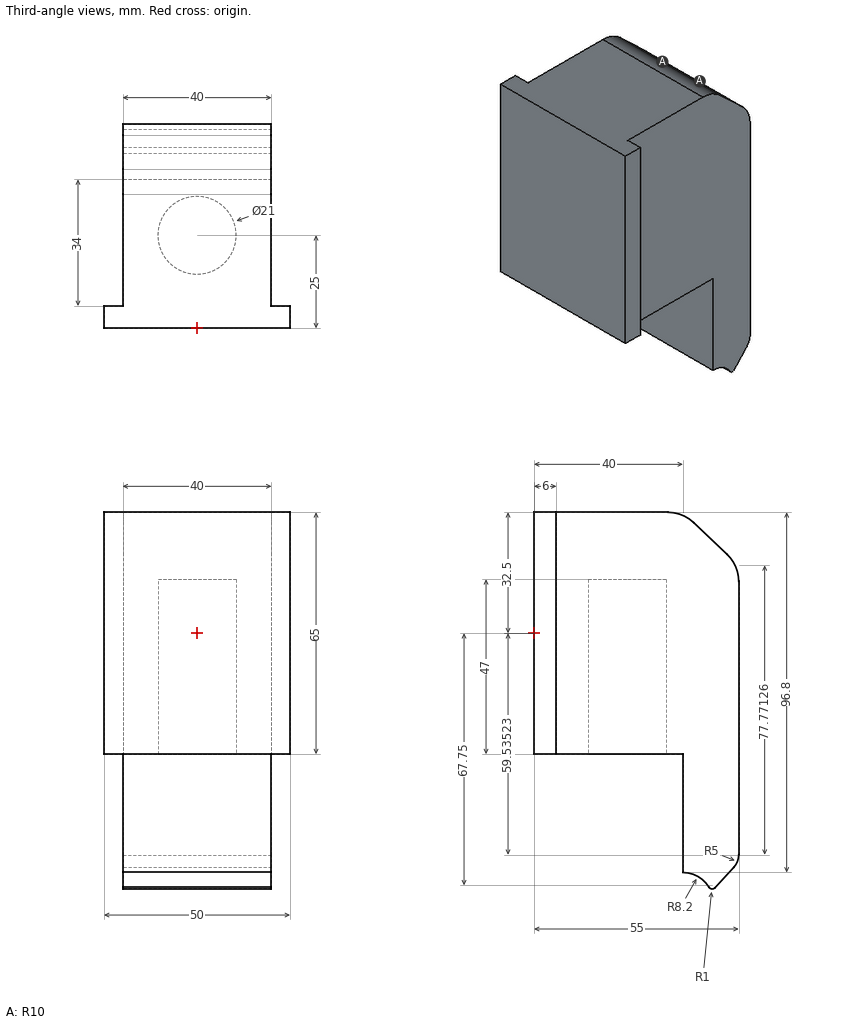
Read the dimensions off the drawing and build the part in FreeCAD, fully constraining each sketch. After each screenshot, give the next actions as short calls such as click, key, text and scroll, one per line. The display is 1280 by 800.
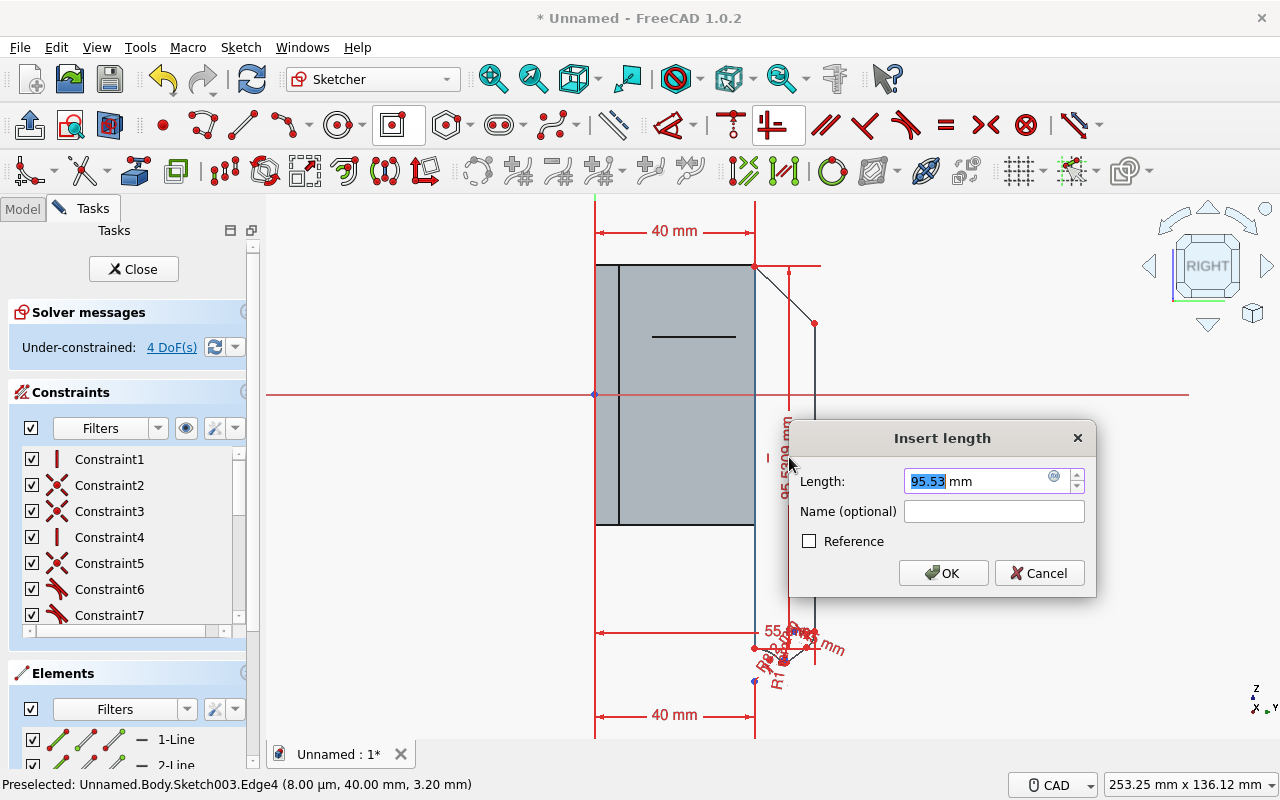
text(96.8)
key(Return)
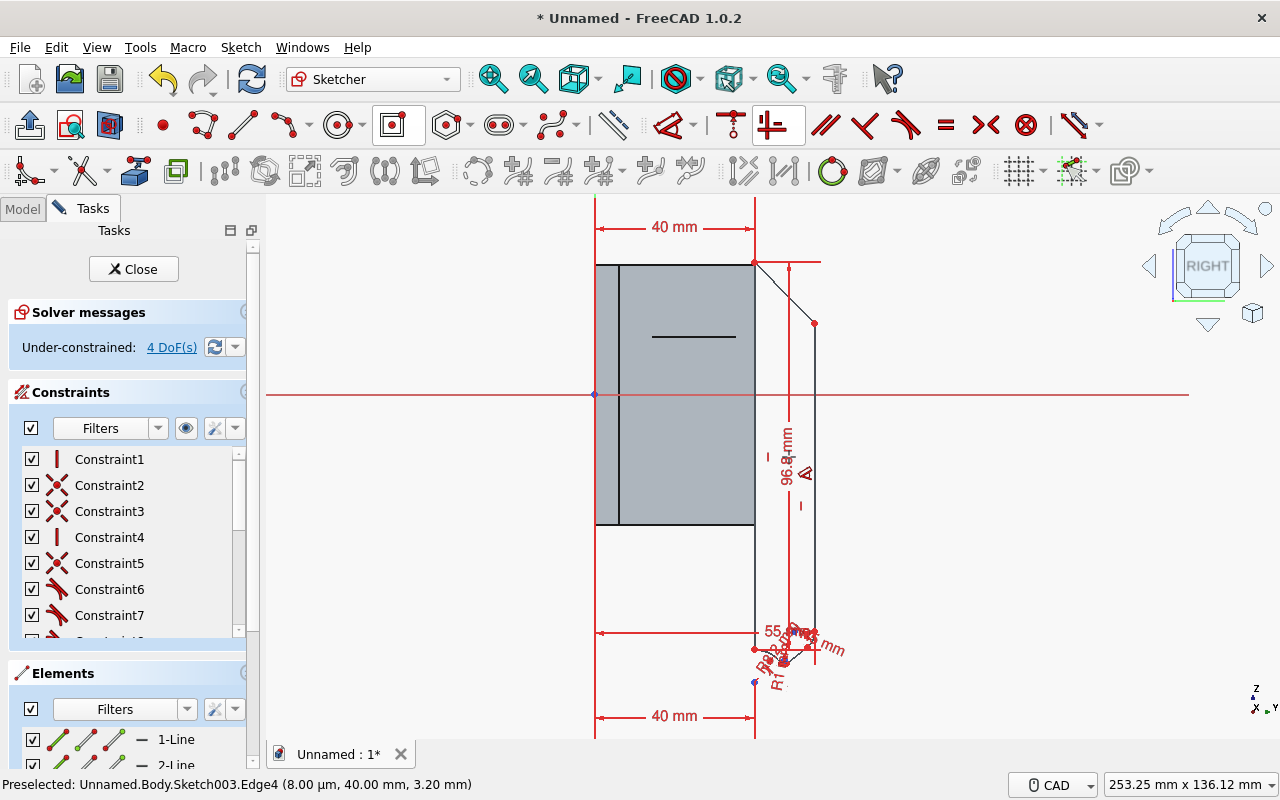
click(755, 262)
click(561, 329)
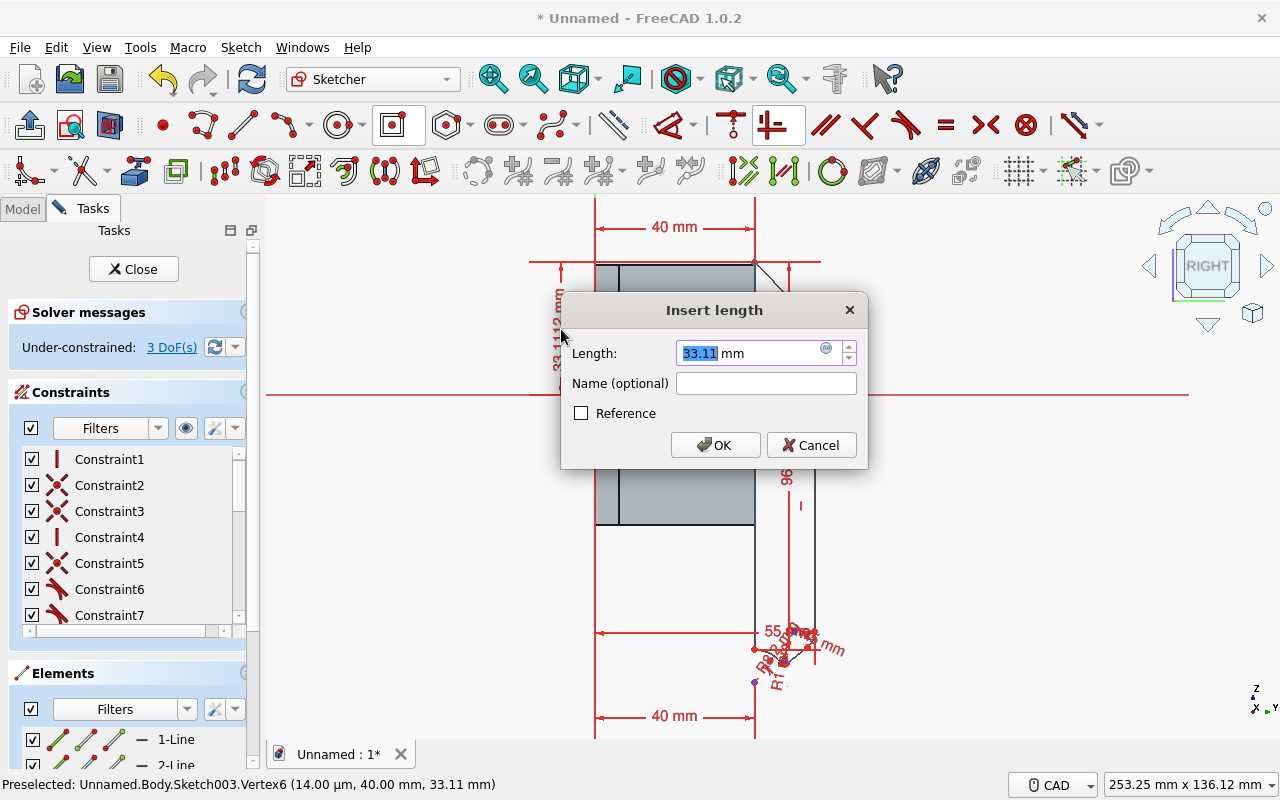
text(32.5)
key(Return)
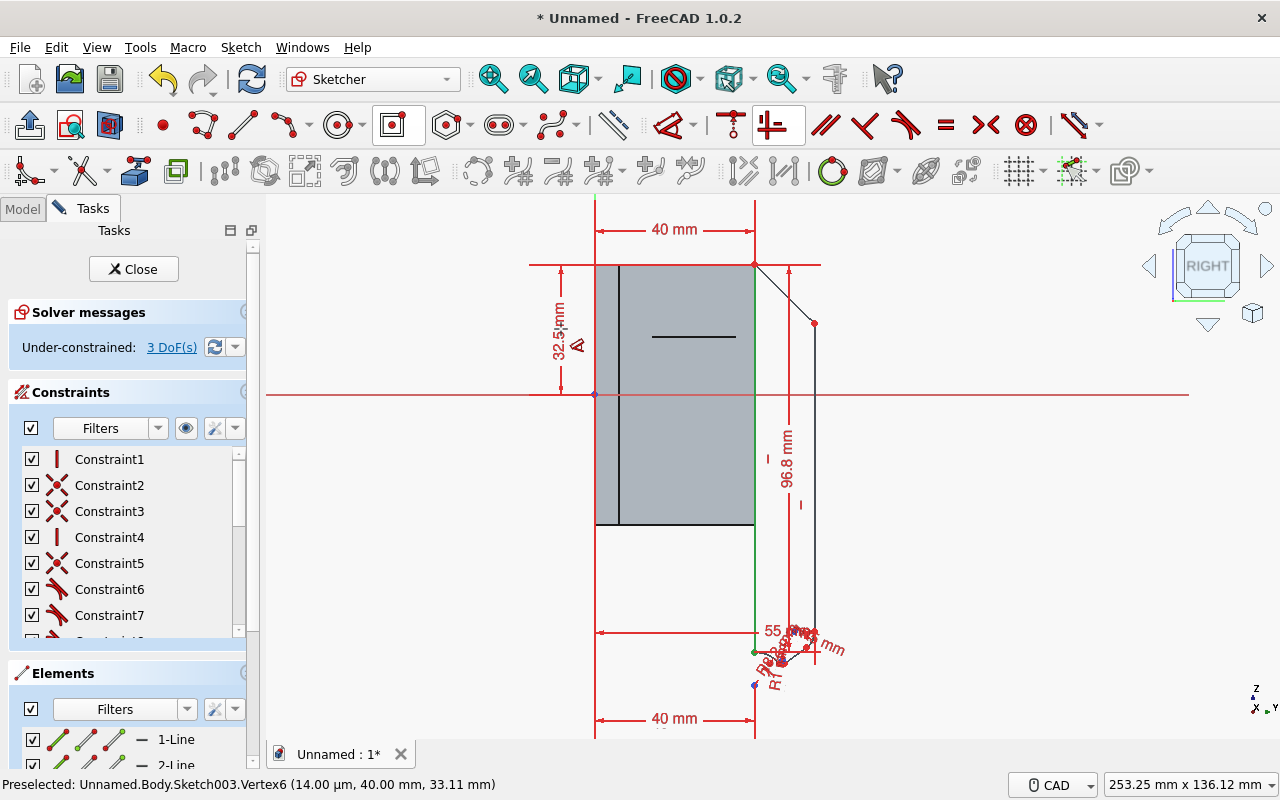
scroll(782, 661, up, 6)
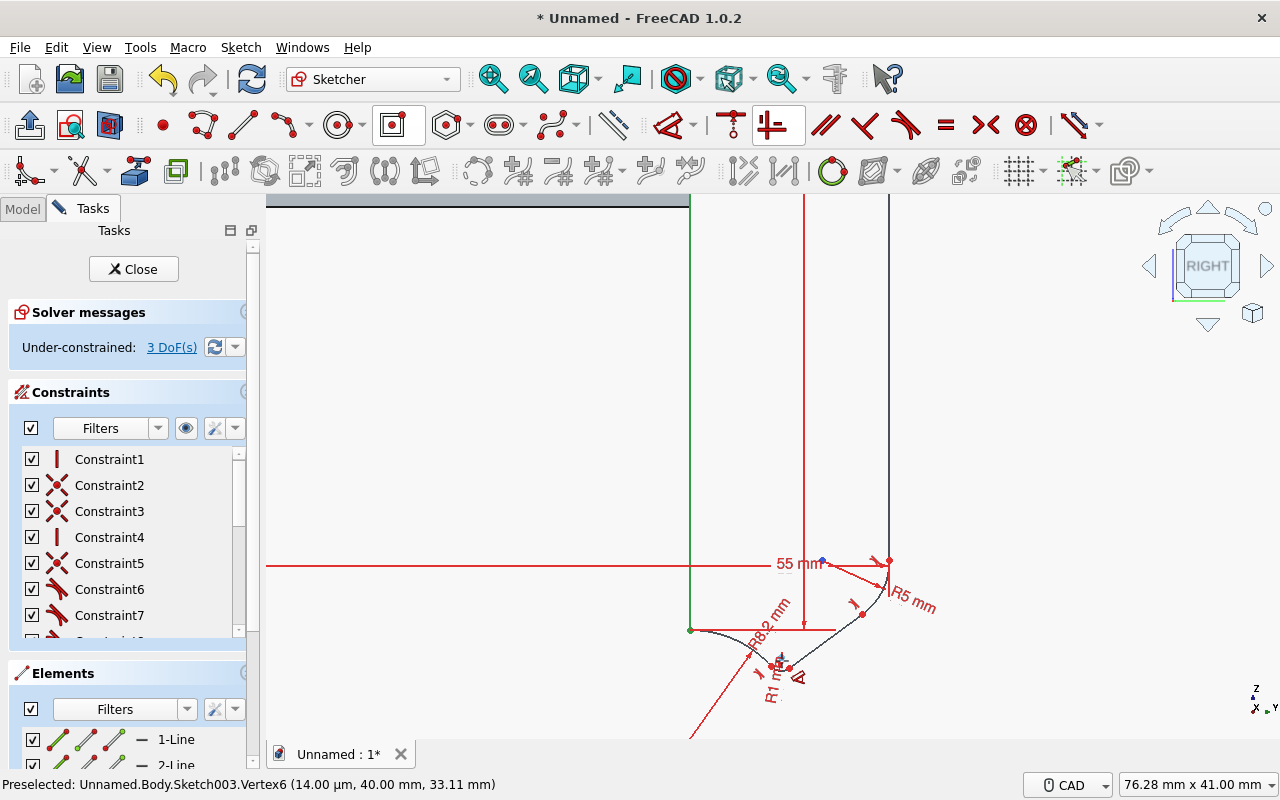
click(781, 658)
click(815, 440)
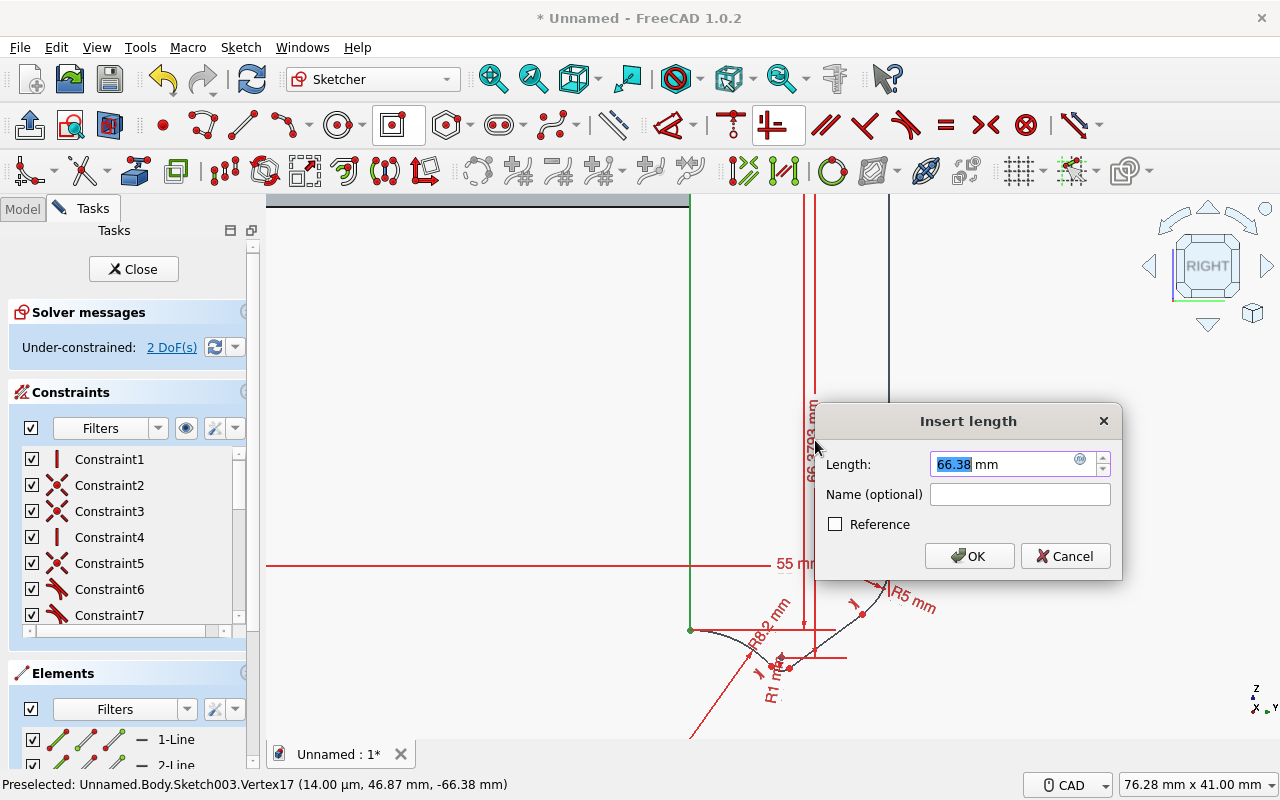
text(67.75)
key(Return)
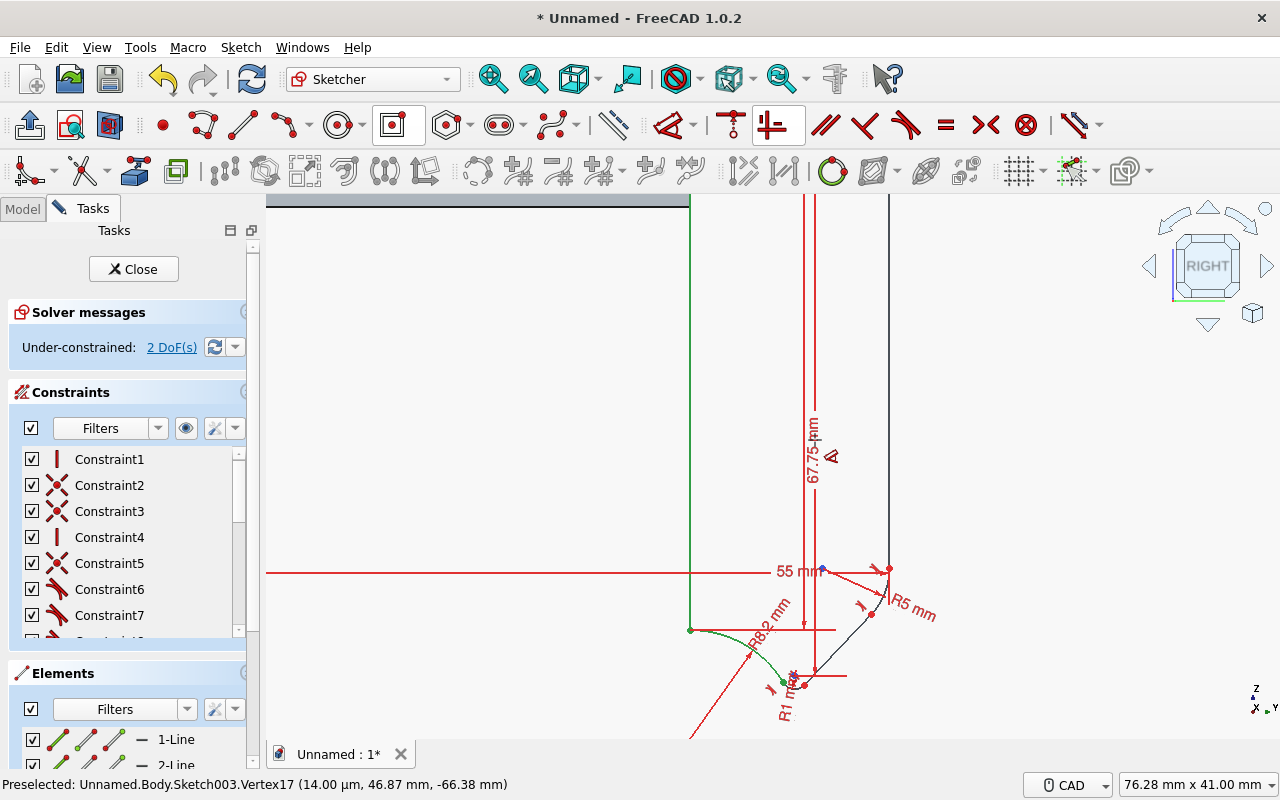
scroll(764, 614, down, 7)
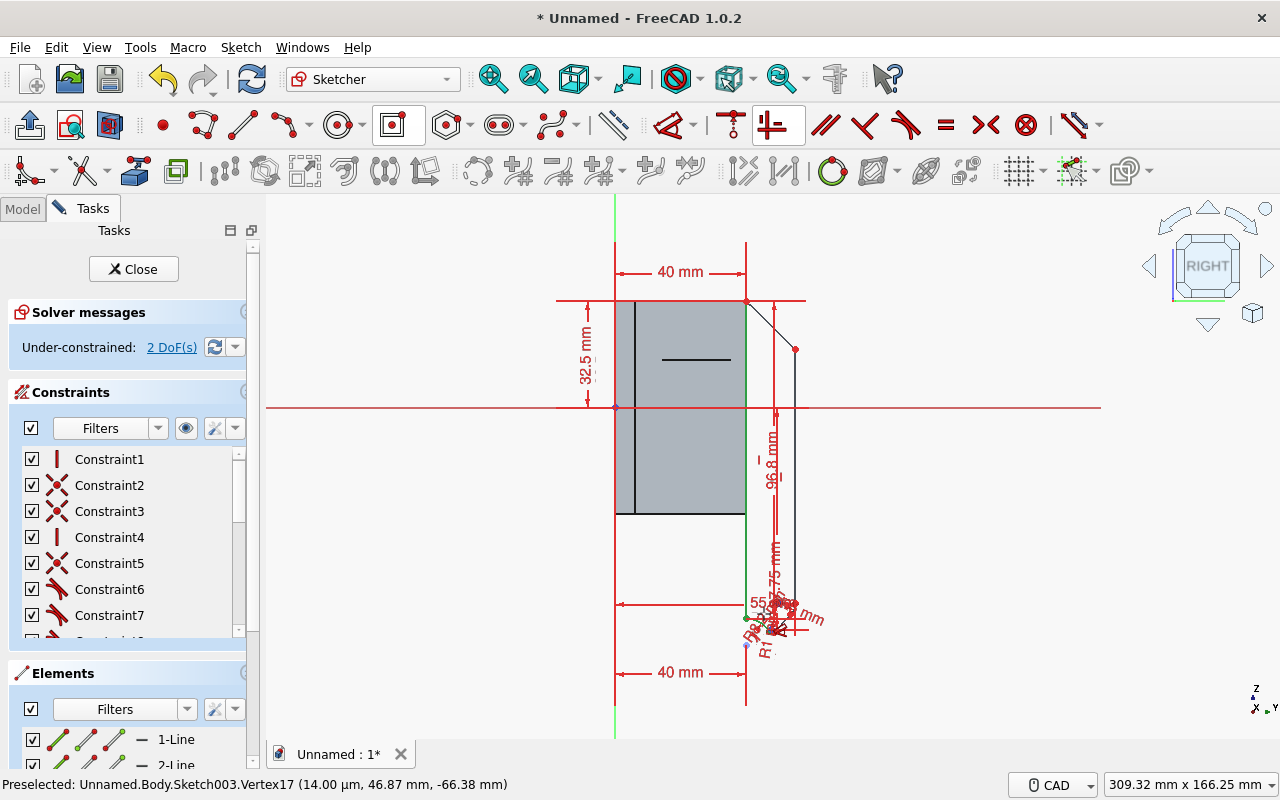
click(795, 527)
click(829, 535)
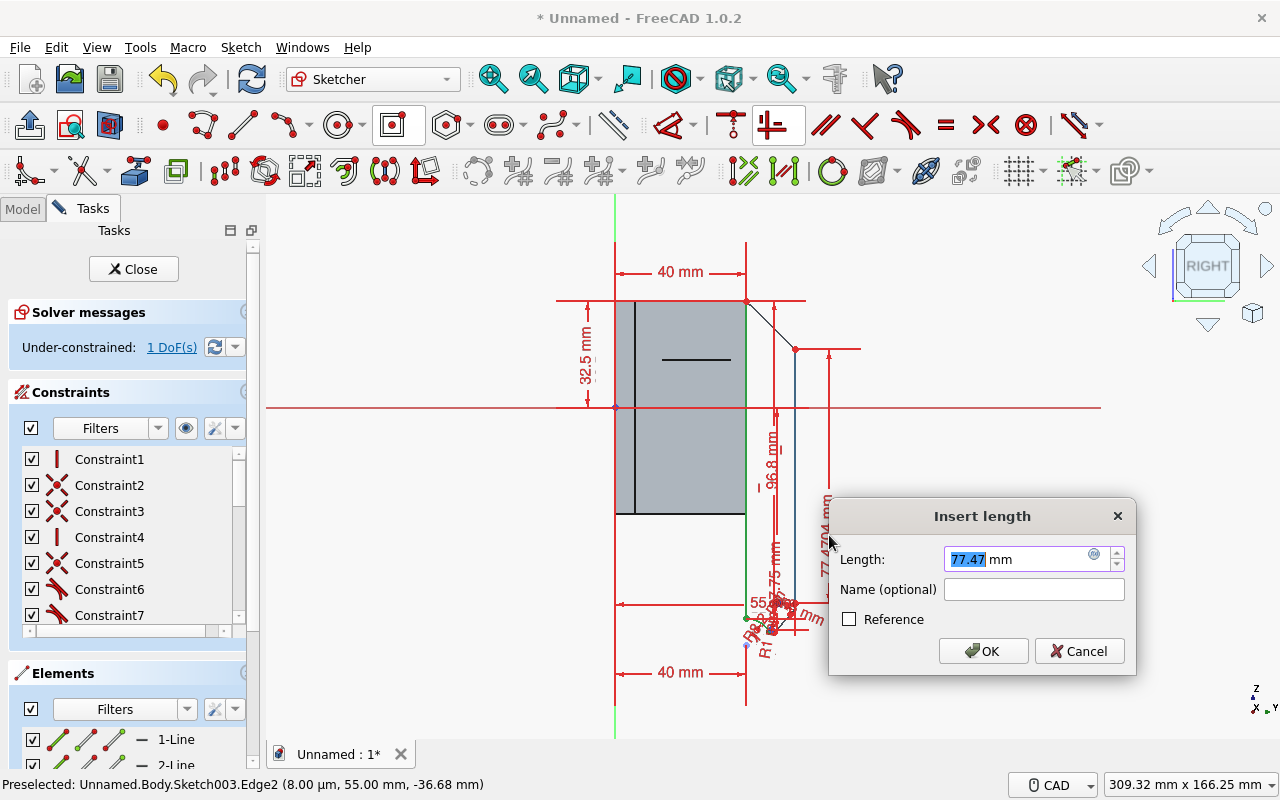
text(77.77126)
key(Return)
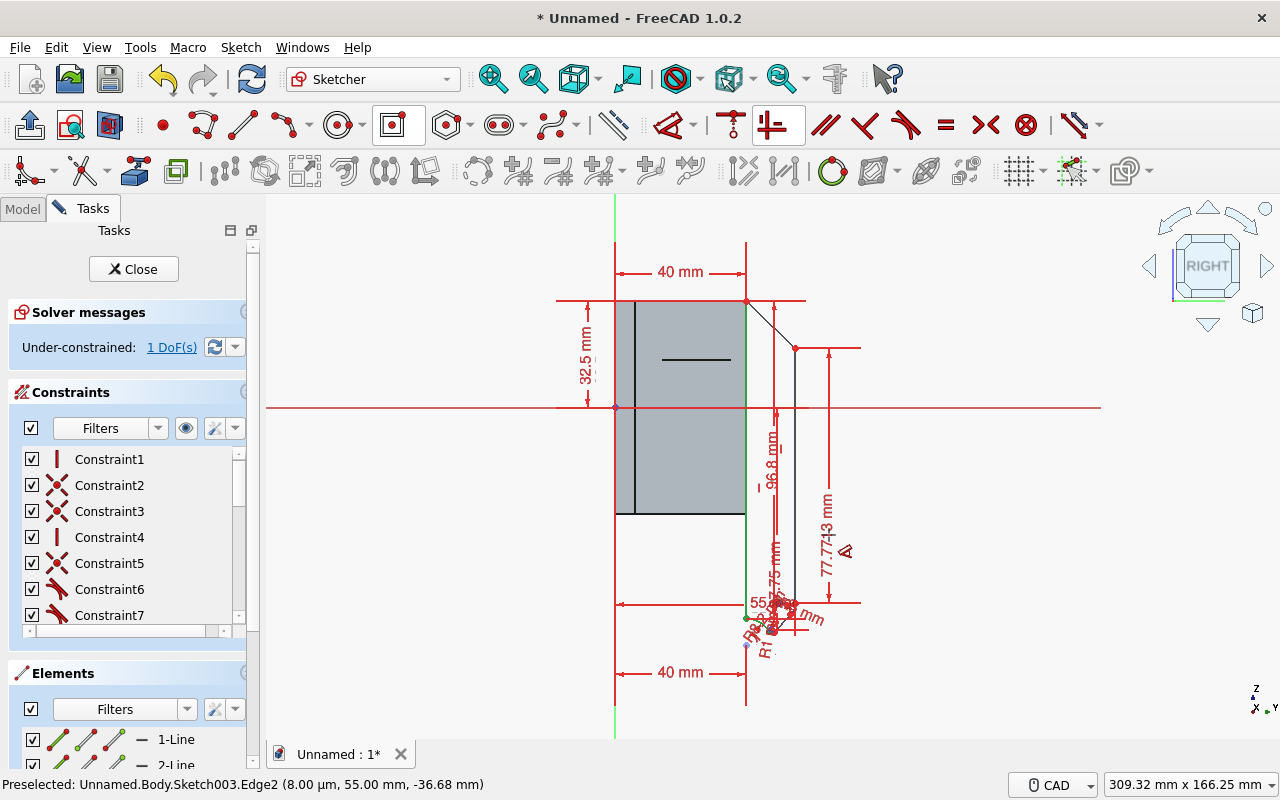
click(795, 603)
click(829, 506)